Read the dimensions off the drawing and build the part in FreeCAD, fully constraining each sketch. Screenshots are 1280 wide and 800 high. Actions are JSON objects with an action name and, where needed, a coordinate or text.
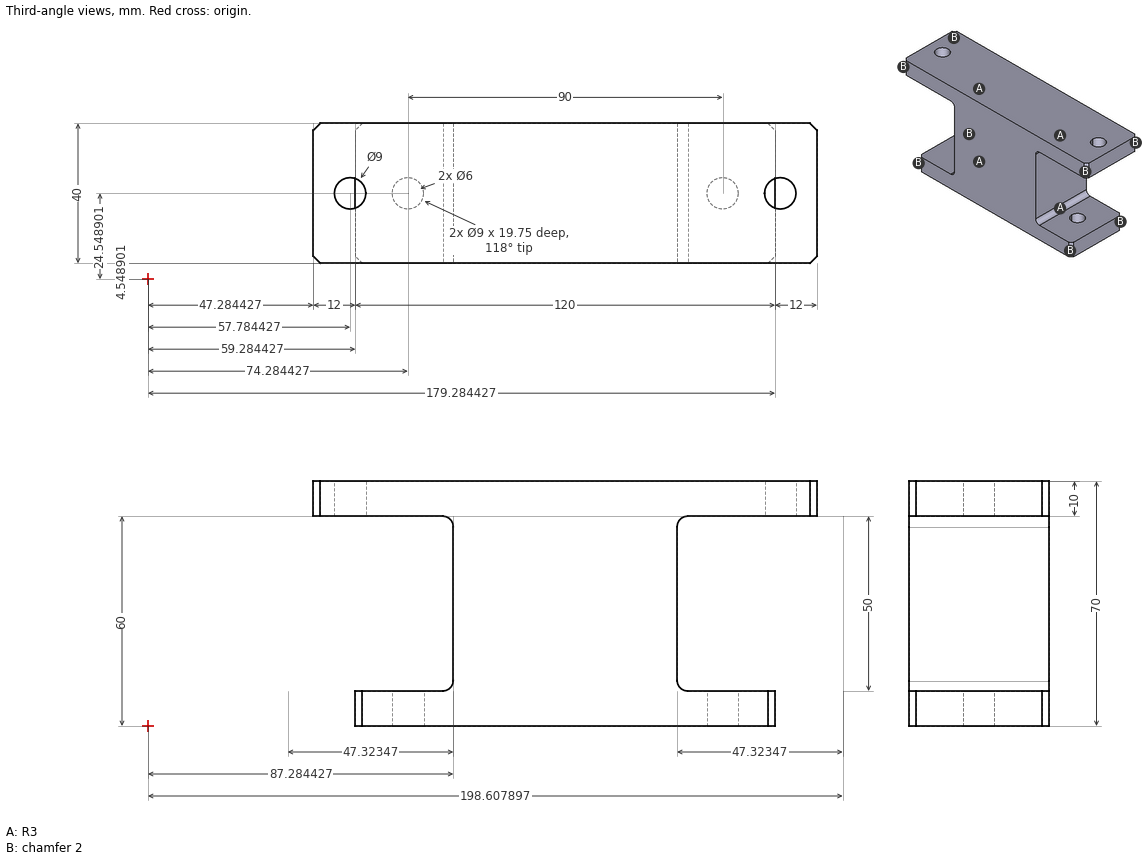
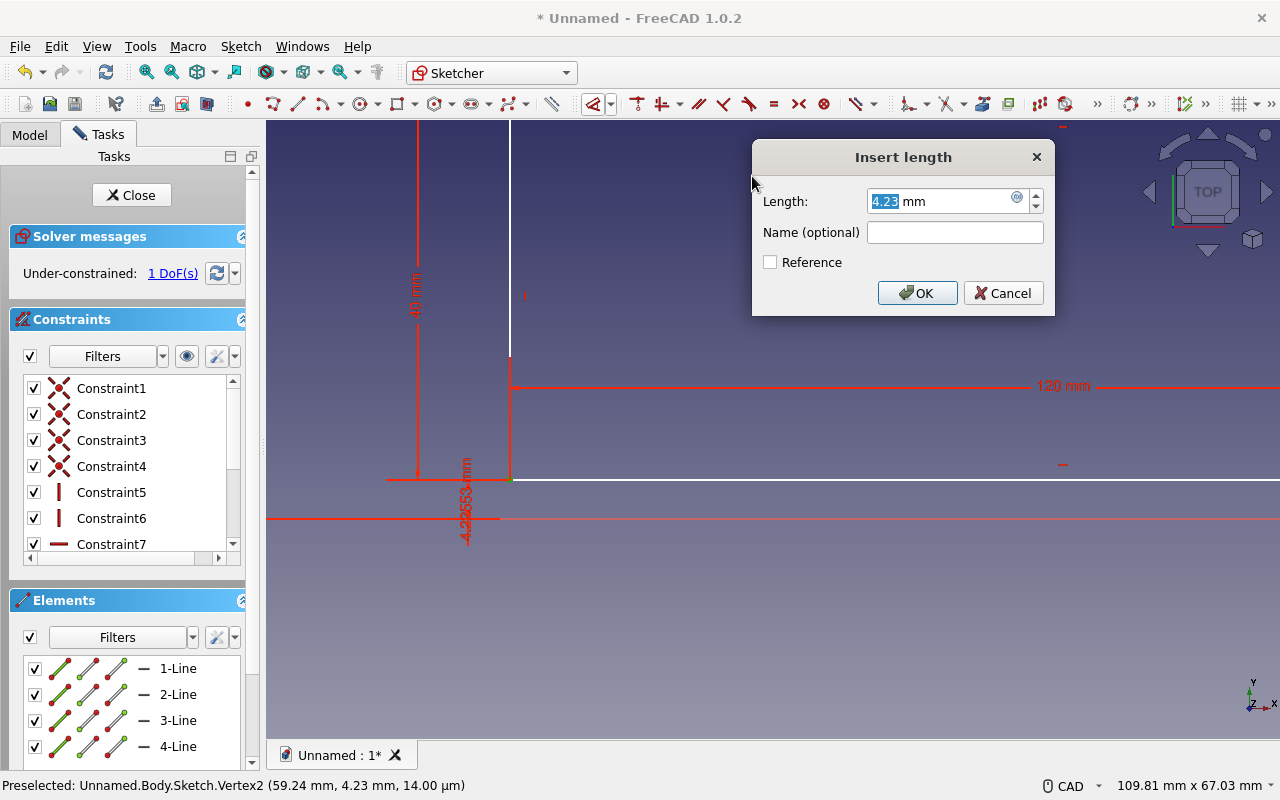
{"action": "type", "text": "4.548901"}
{"action": "key", "text": "Return"}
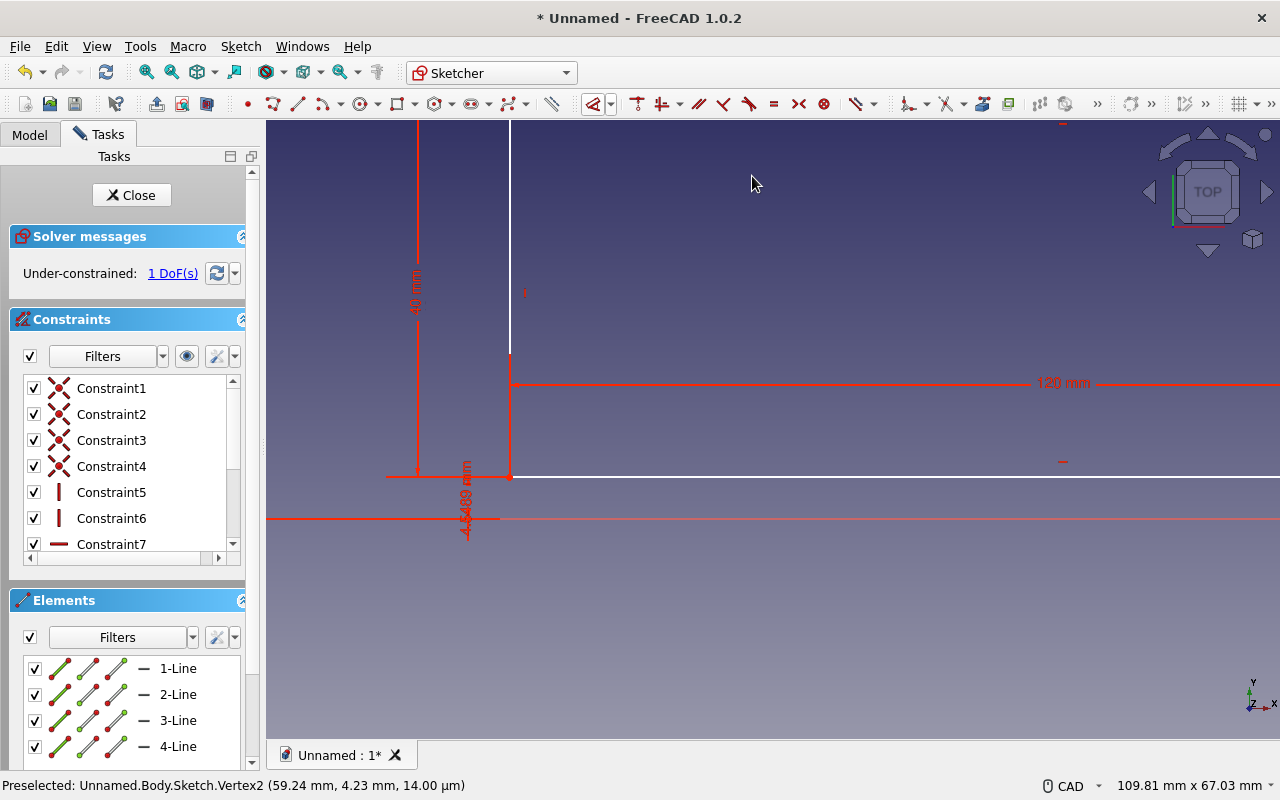
{"action": "scroll", "coordinate": [655, 497], "scroll_direction": "down", "scroll_amount": 5}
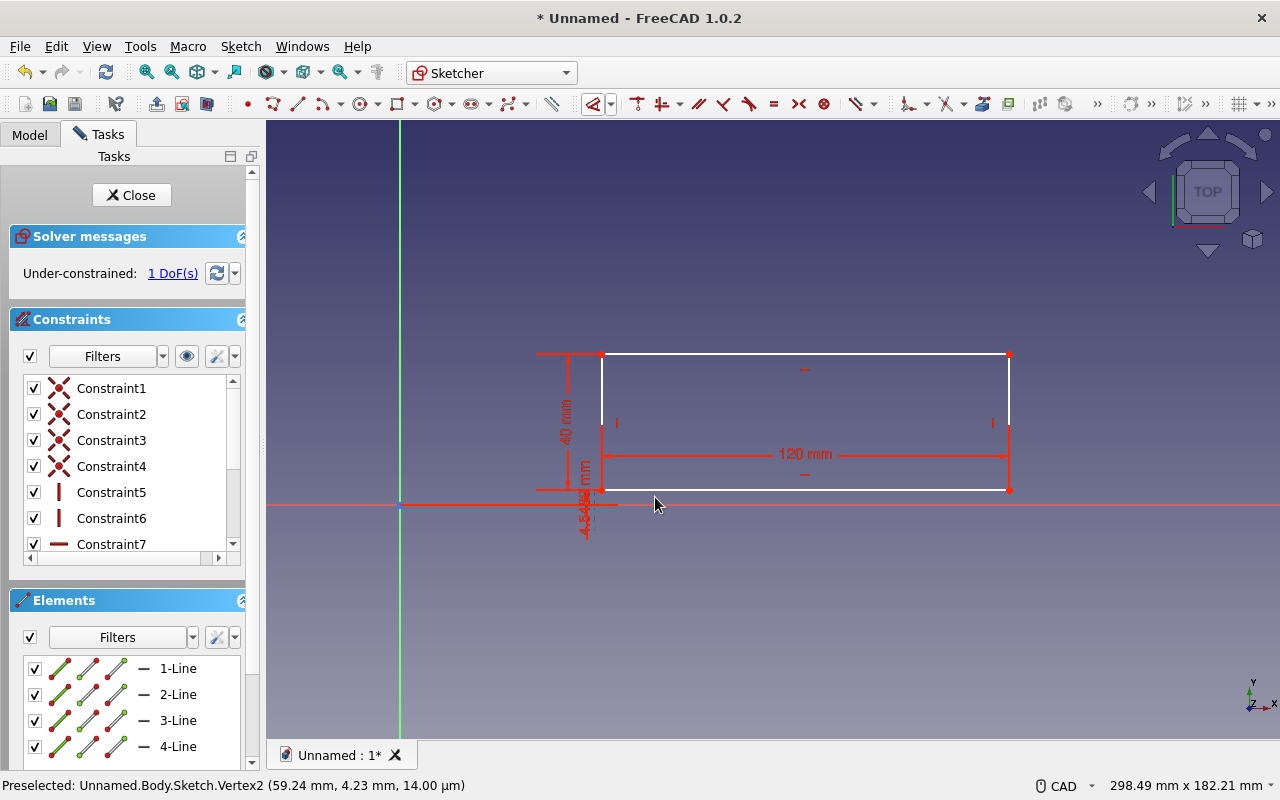
{"action": "left_click", "coordinate": [602, 354]}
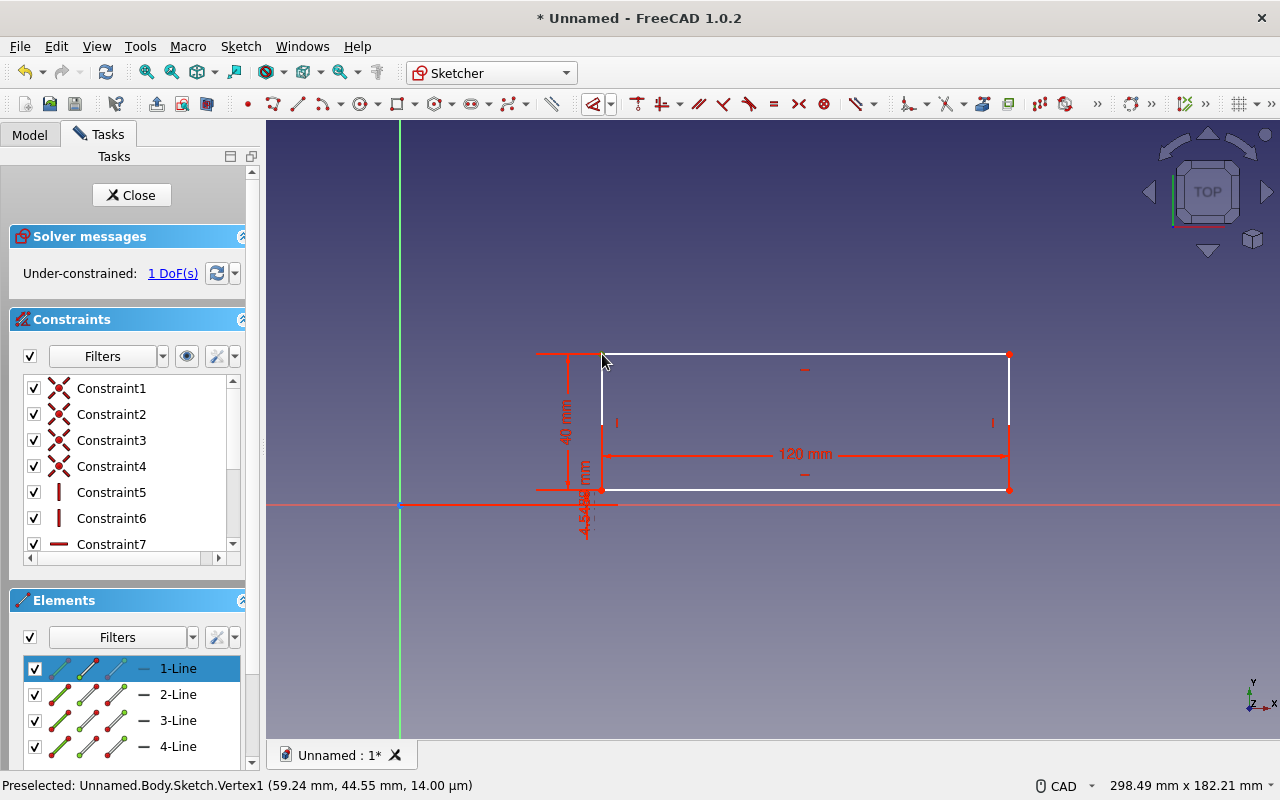
{"action": "key", "text": "l"}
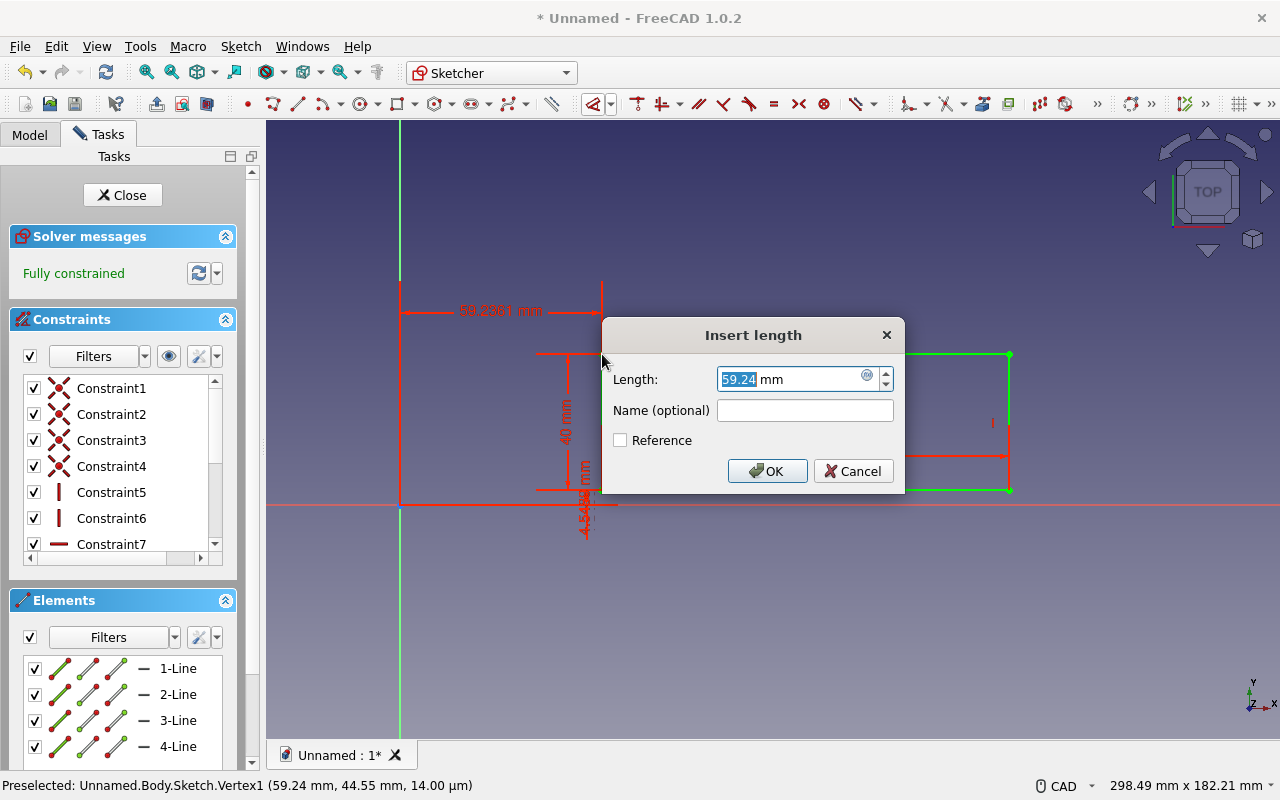
{"action": "type", "text": "59.284427"}
{"action": "key", "text": "Return"}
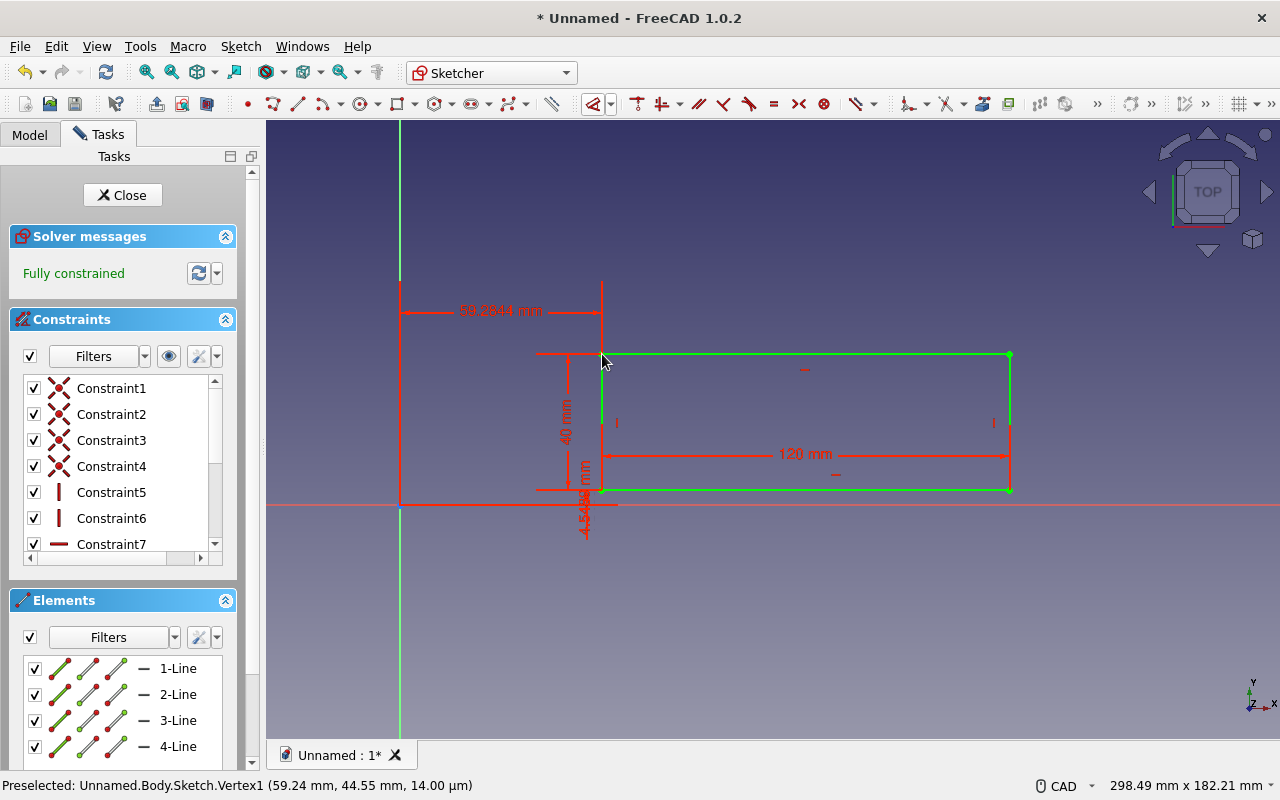
{"action": "left_click", "coordinate": [123, 195]}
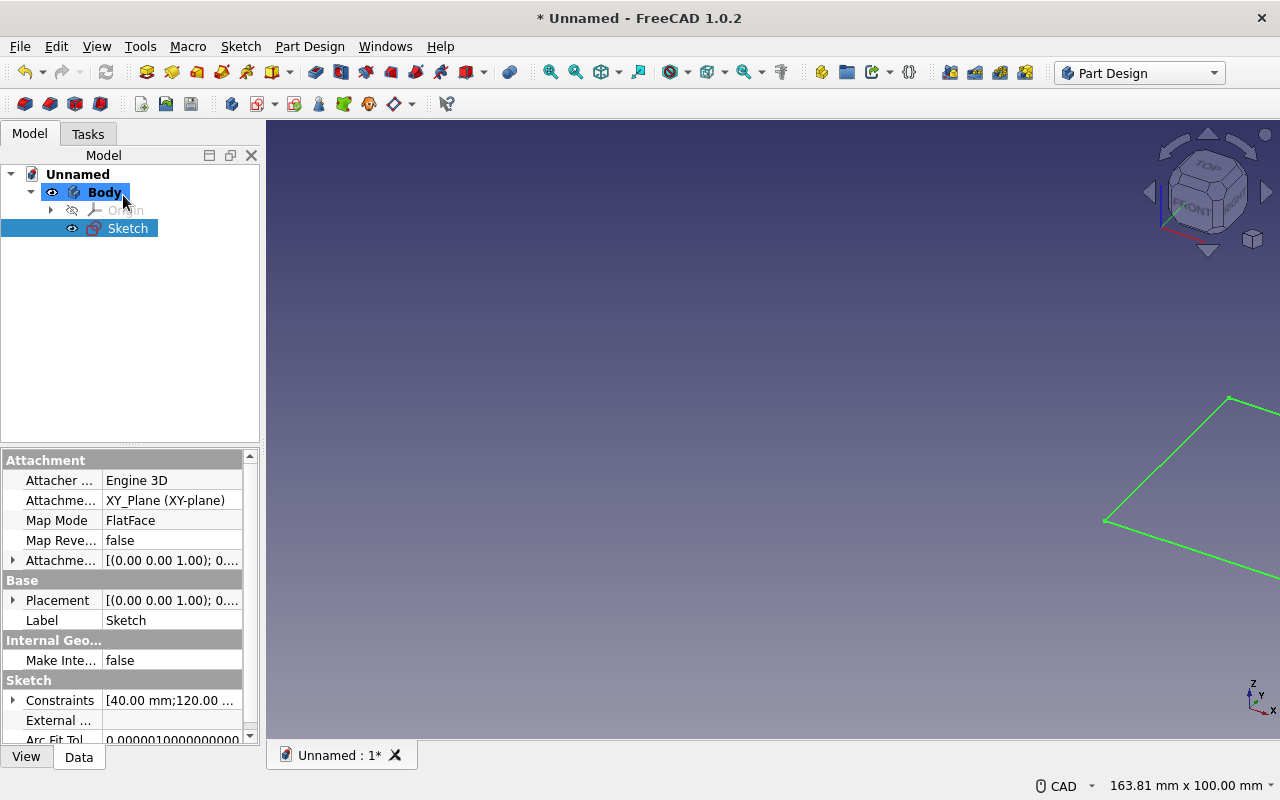
{"action": "left_click", "coordinate": [147, 72]}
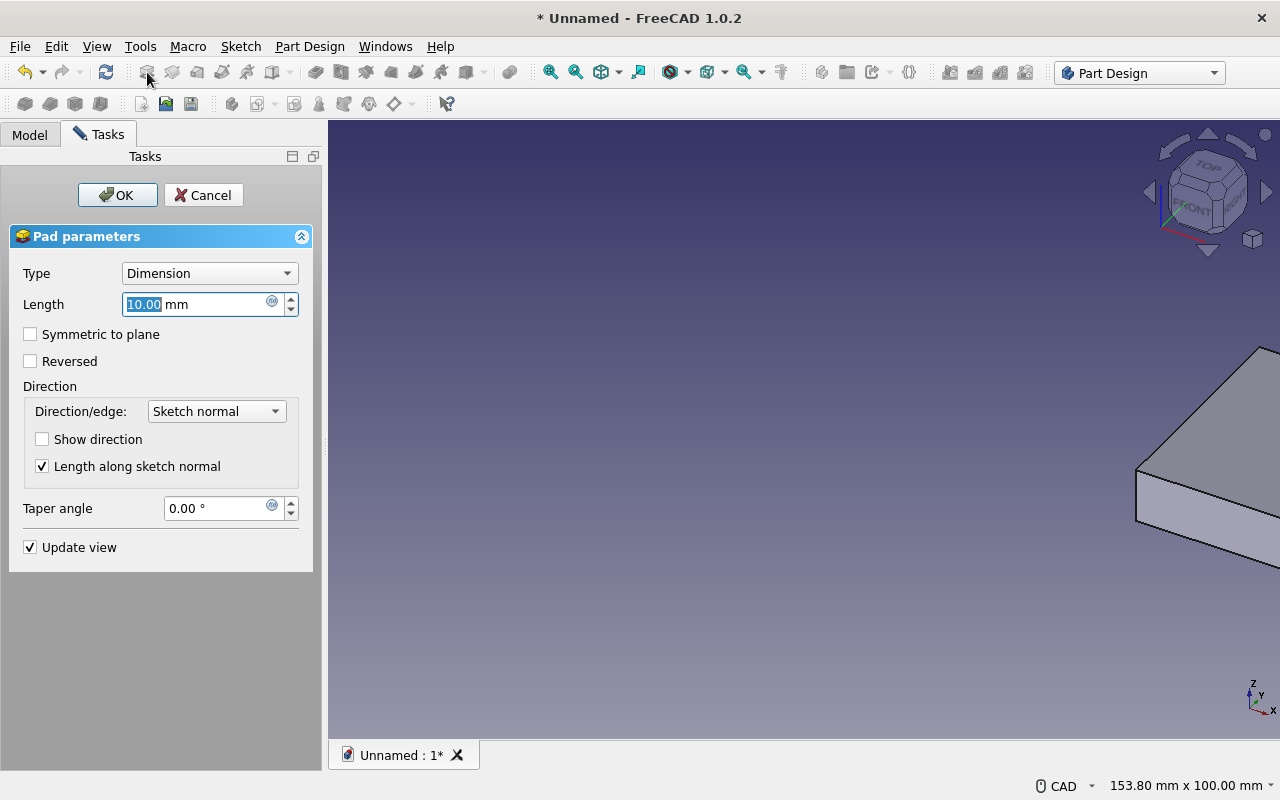
{"action": "type", "text": "70"}
{"action": "key", "text": "Tab"}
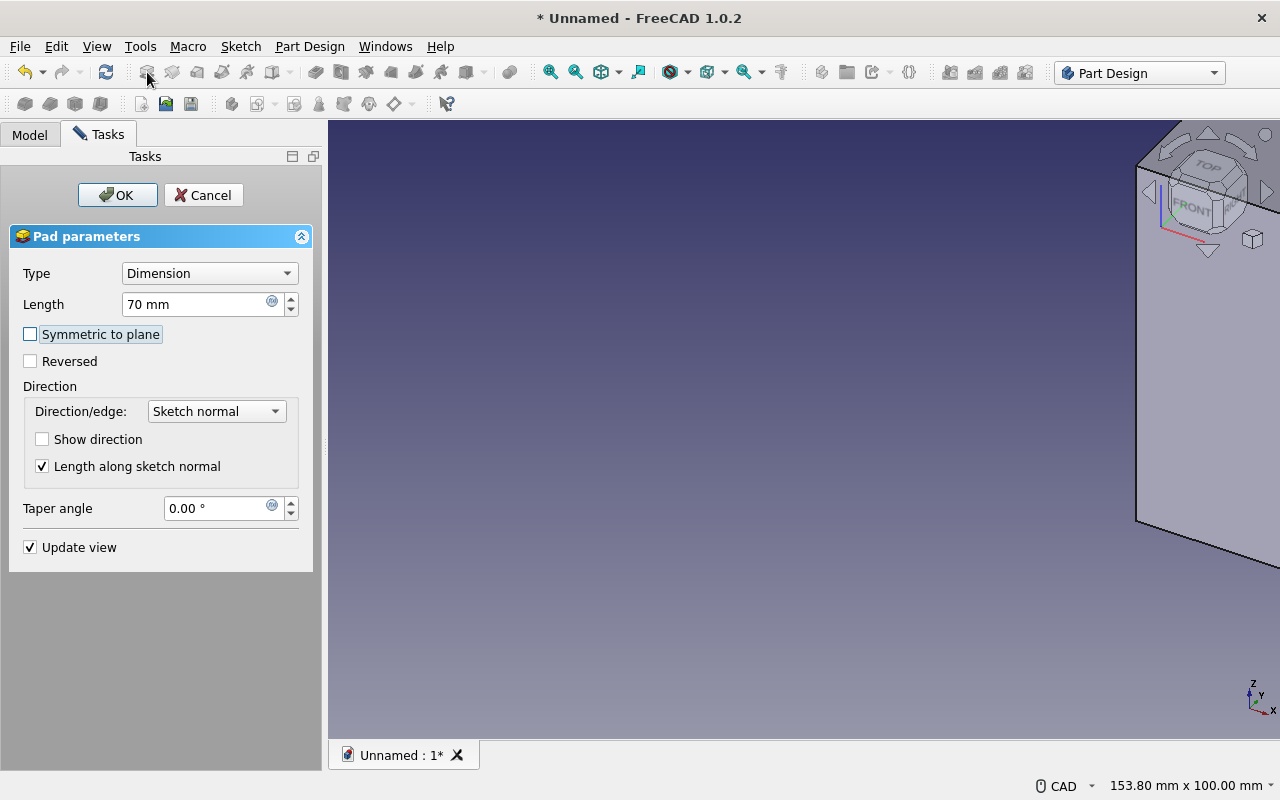
{"action": "left_click", "coordinate": [118, 195]}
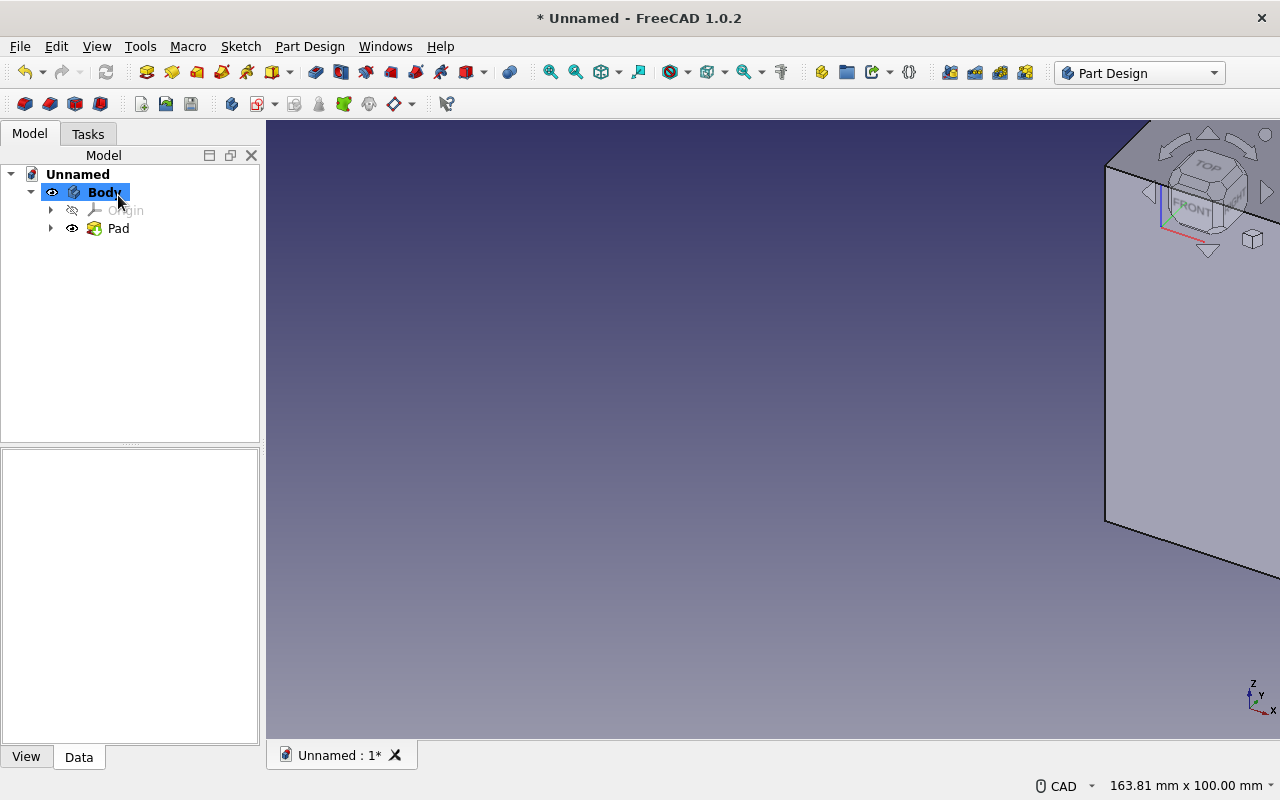
{"action": "left_click", "coordinate": [551, 72]}